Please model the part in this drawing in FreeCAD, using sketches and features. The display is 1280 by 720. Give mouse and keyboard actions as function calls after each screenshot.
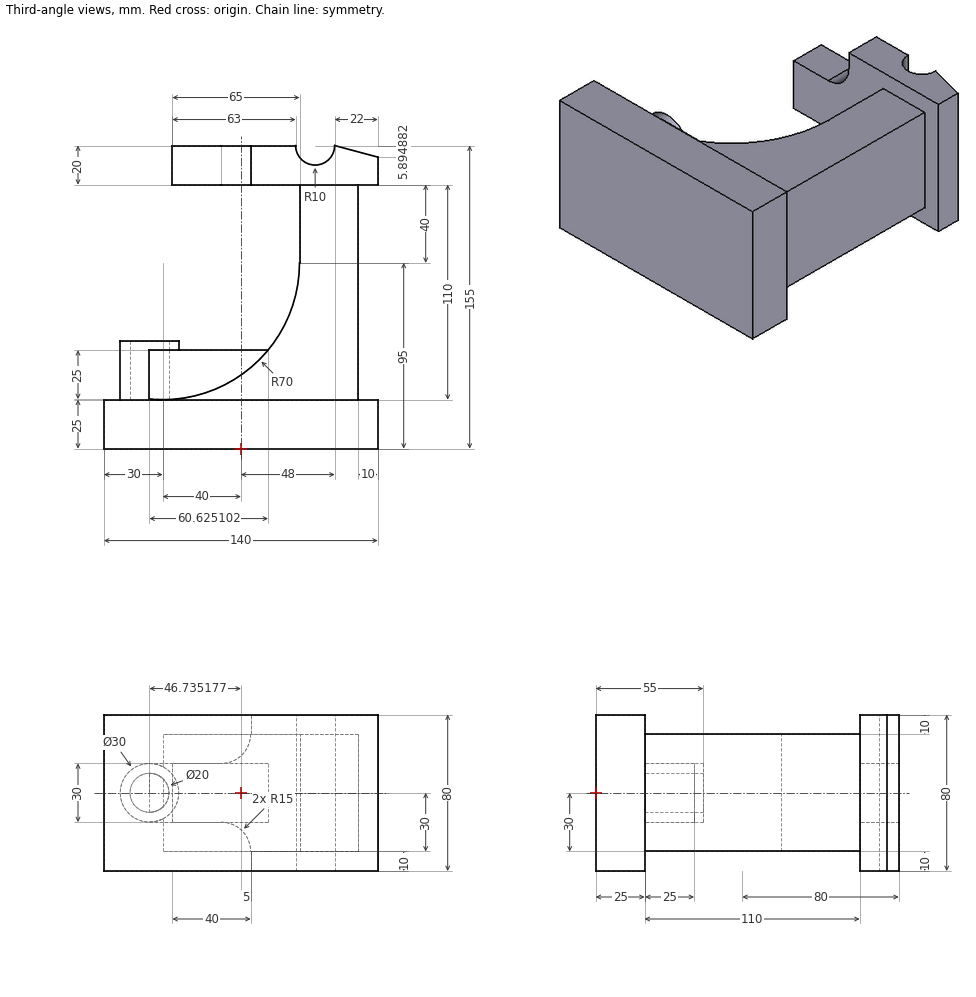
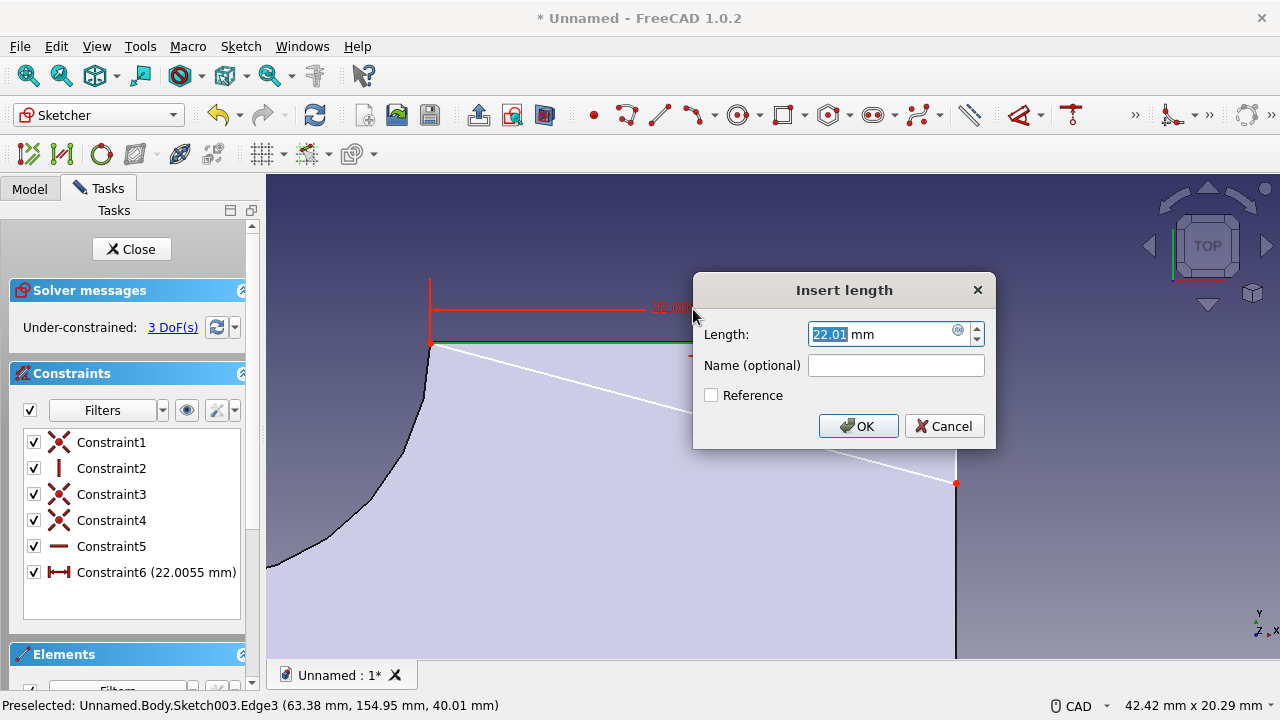
text(22)
key(Return)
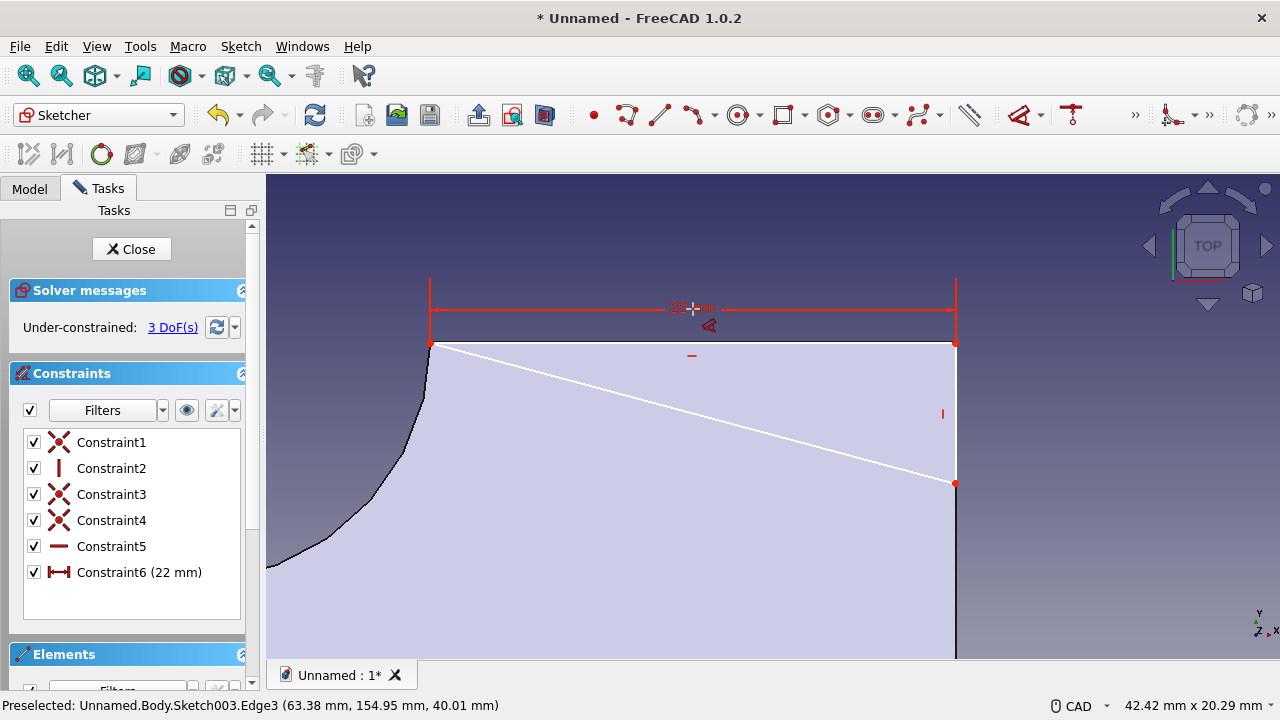
click(430, 343)
click(362, 309)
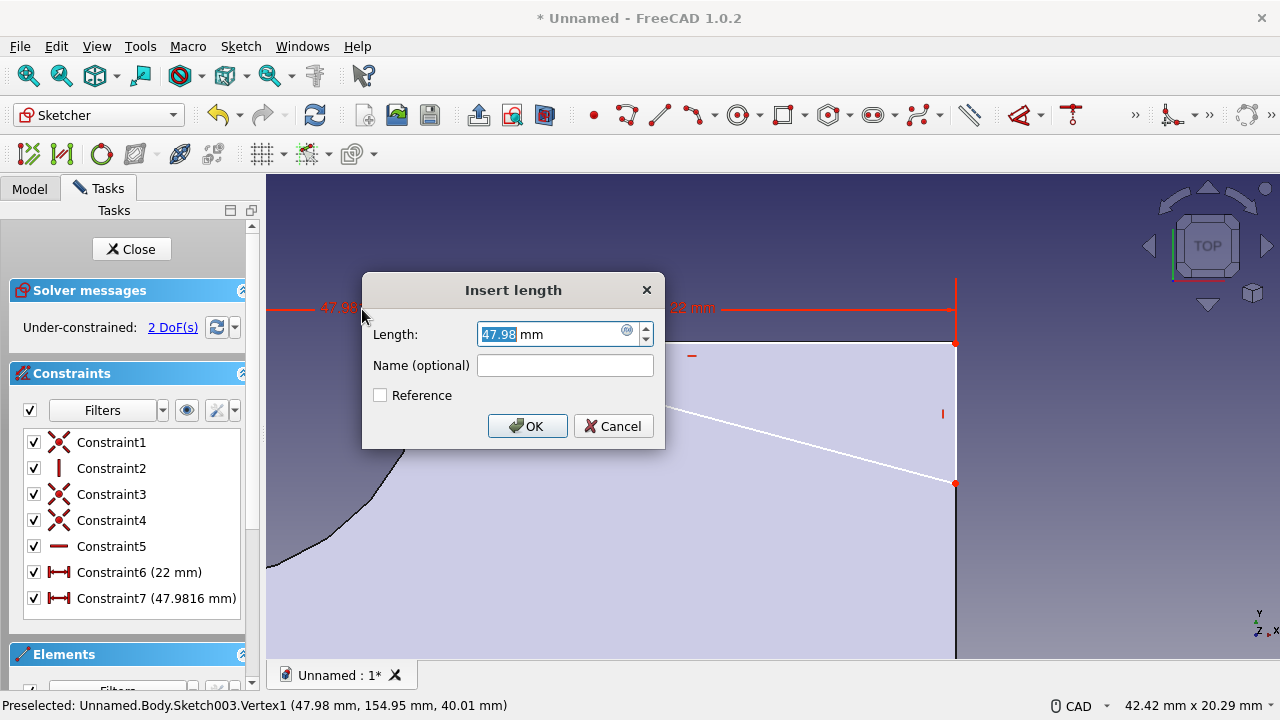
text(48)
key(Return)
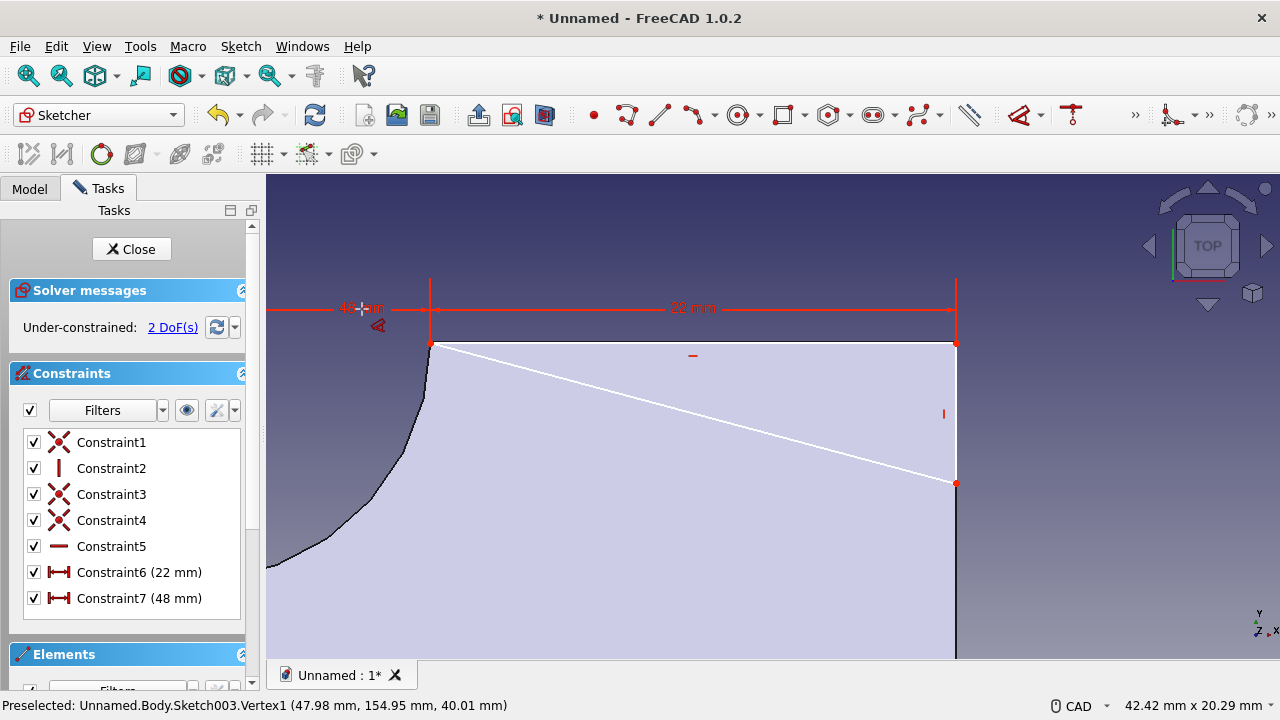
click(430, 343)
click(464, 487)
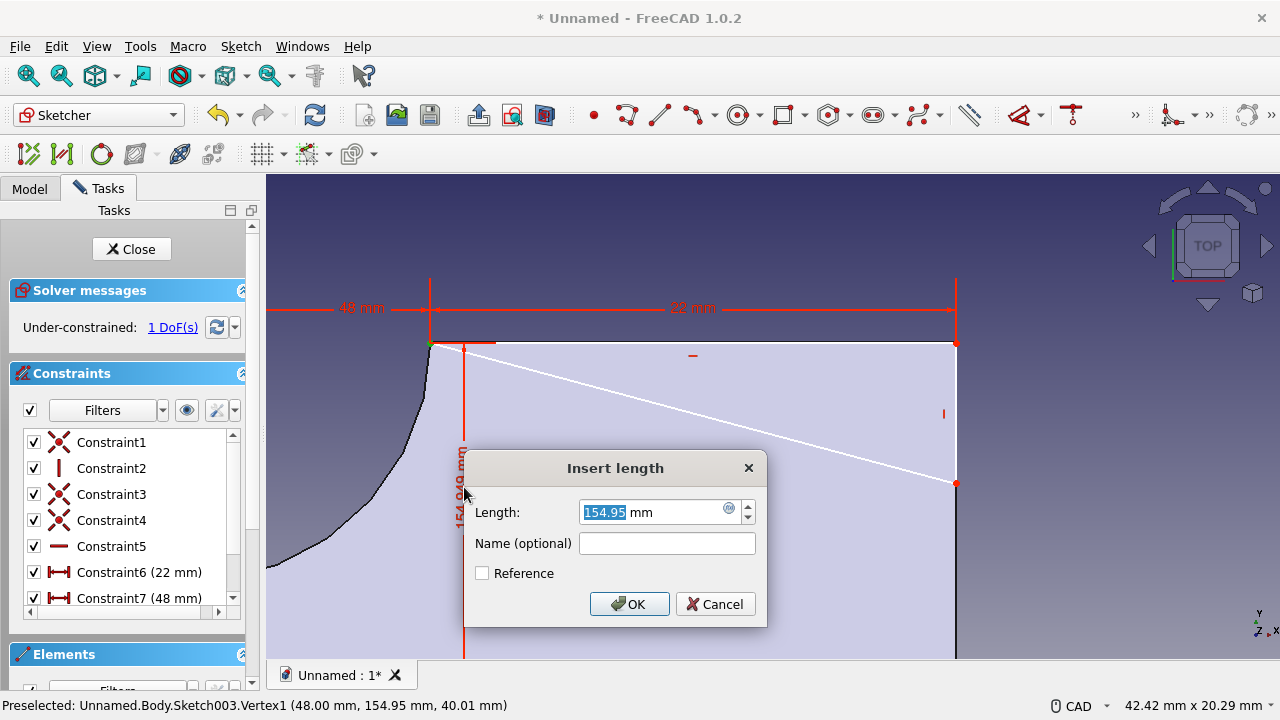
text(155)
key(Return)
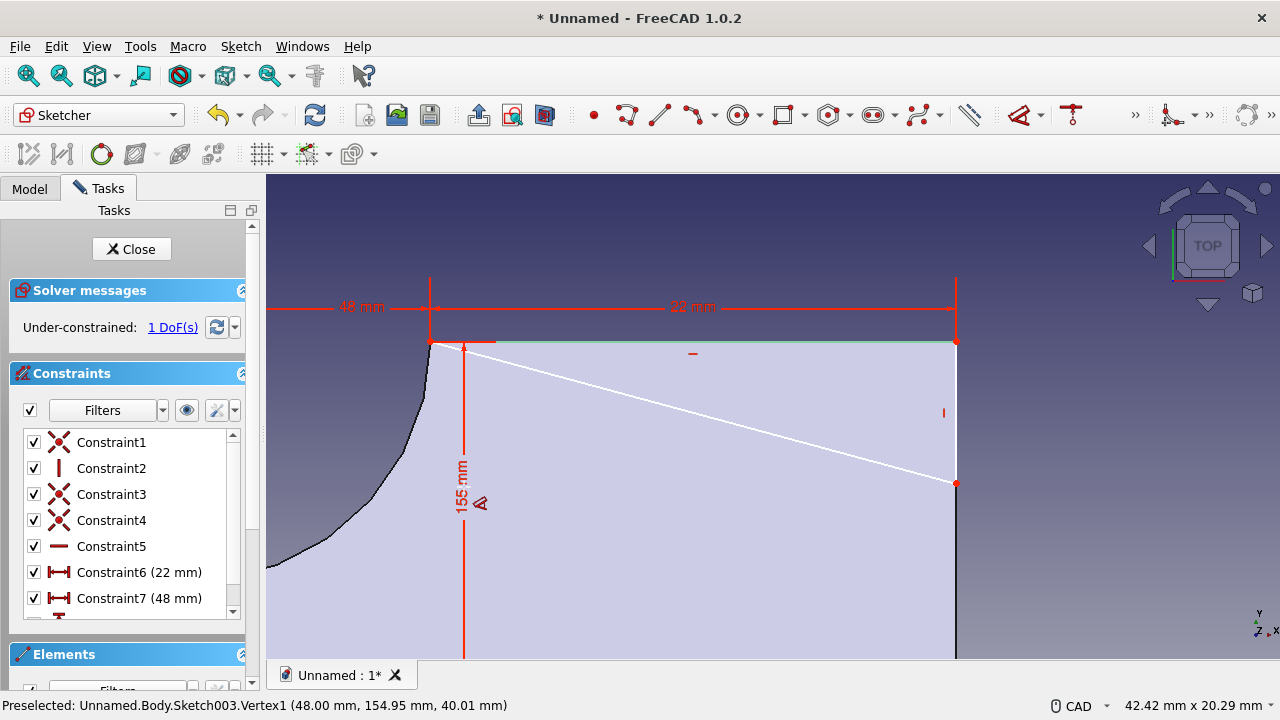
click(956, 441)
click(990, 413)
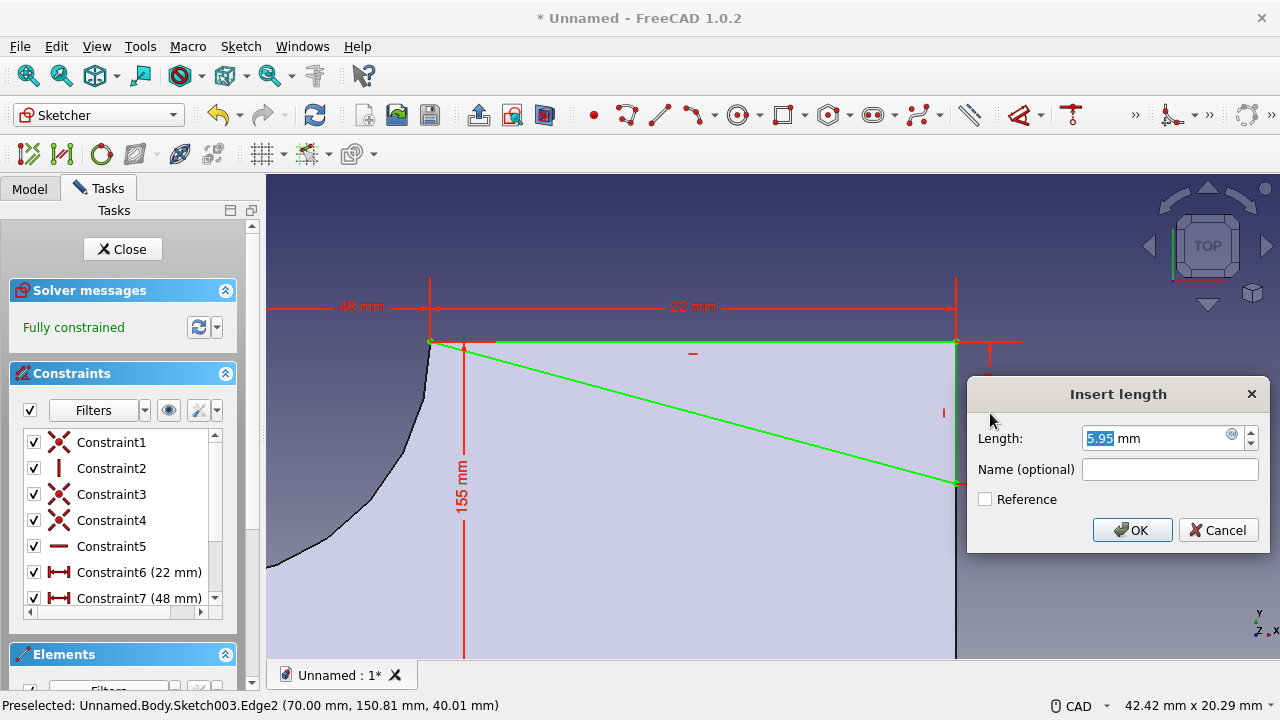
text(5.894882)
key(Return)
key(Escape)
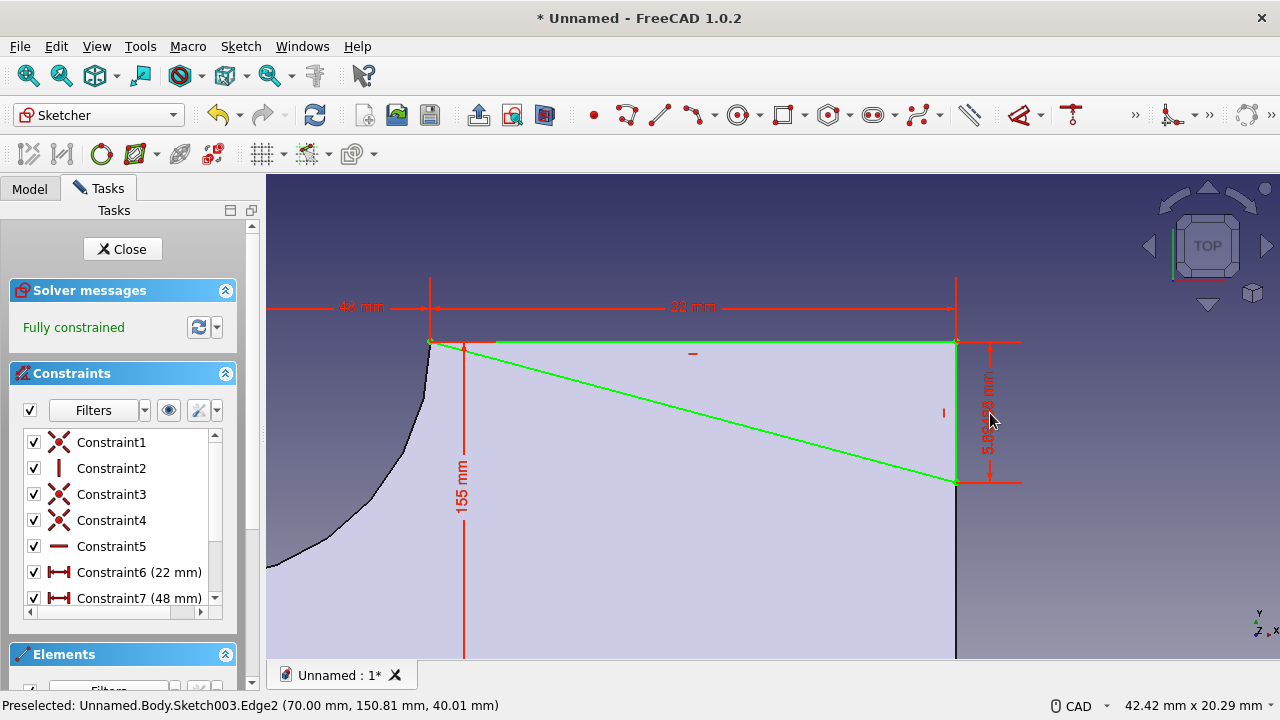
click(123, 249)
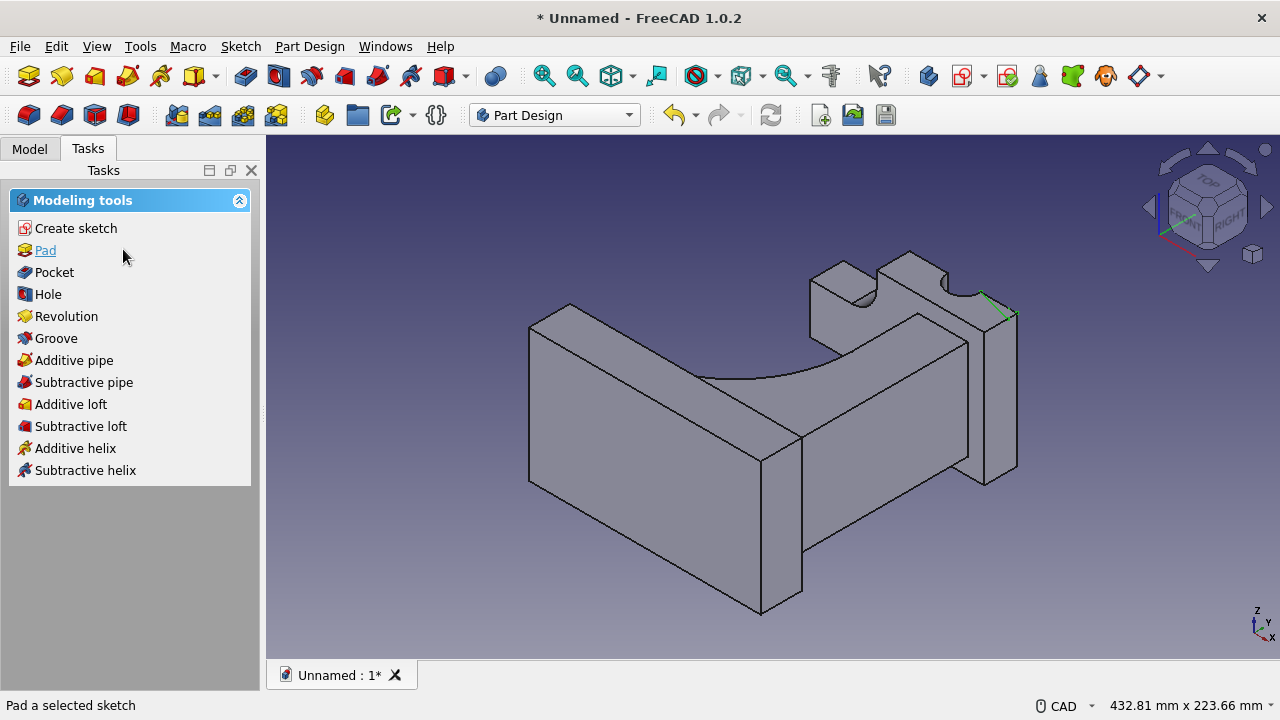
click(246, 76)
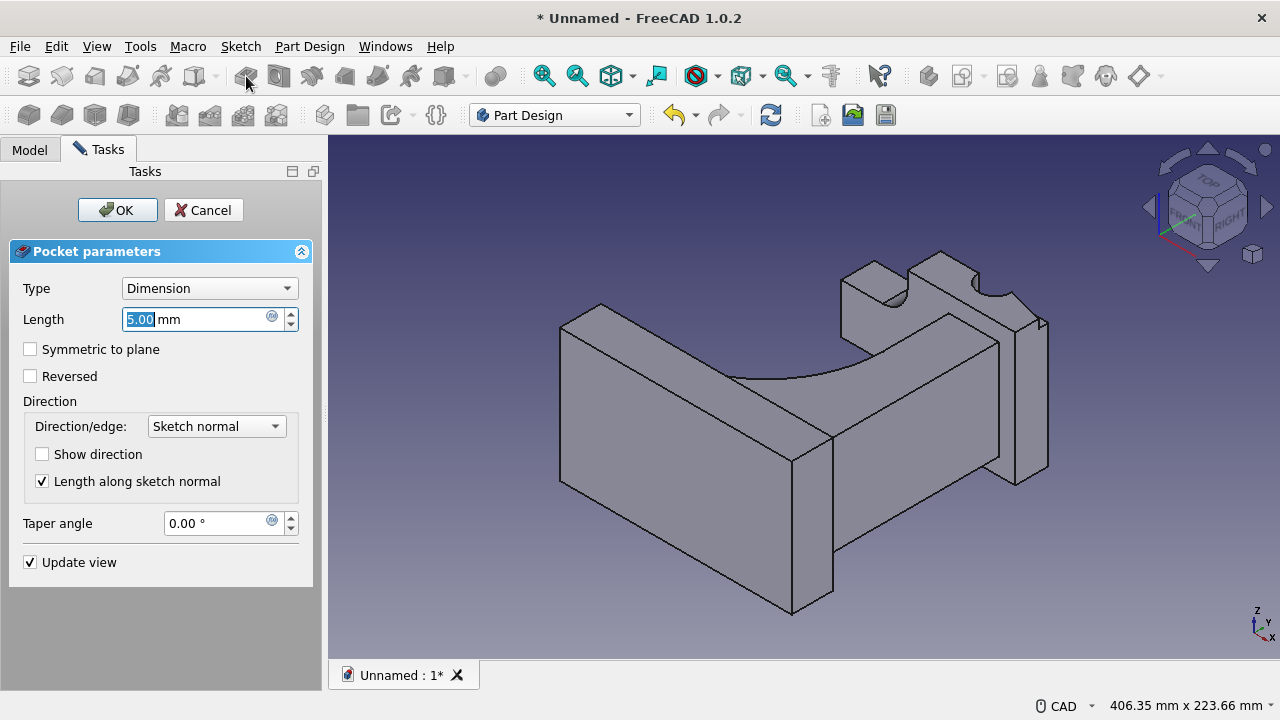
text(80)
key(Tab)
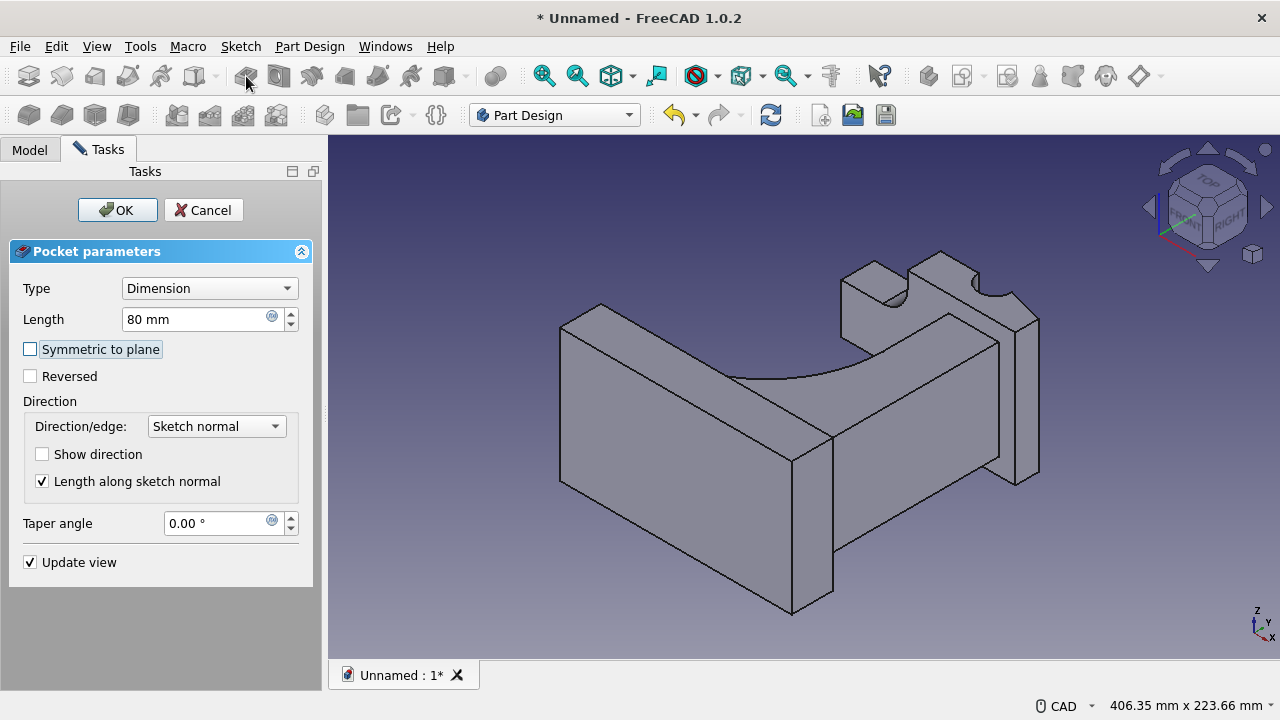
click(118, 210)